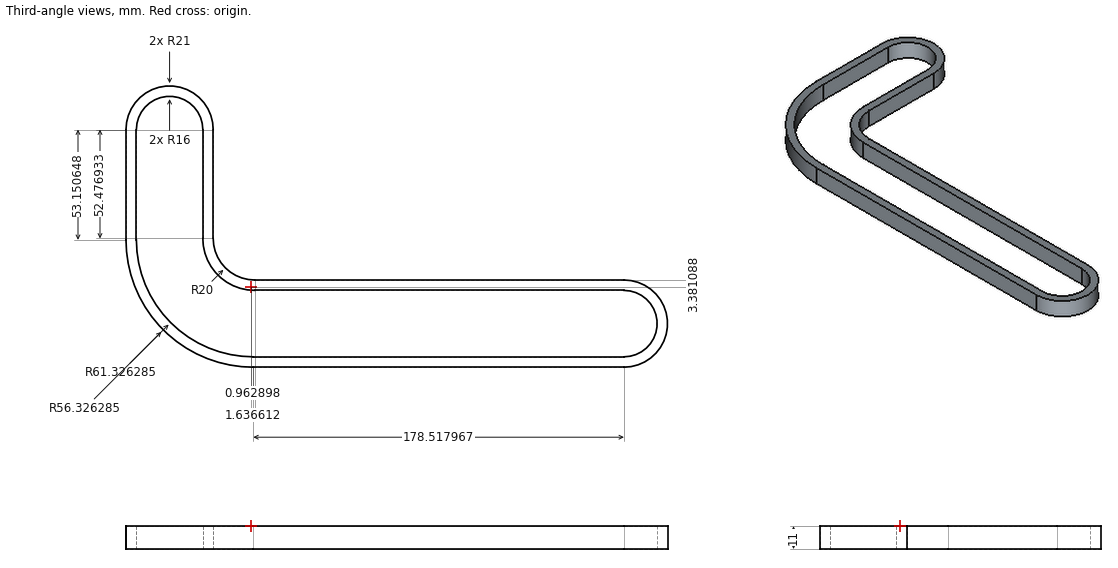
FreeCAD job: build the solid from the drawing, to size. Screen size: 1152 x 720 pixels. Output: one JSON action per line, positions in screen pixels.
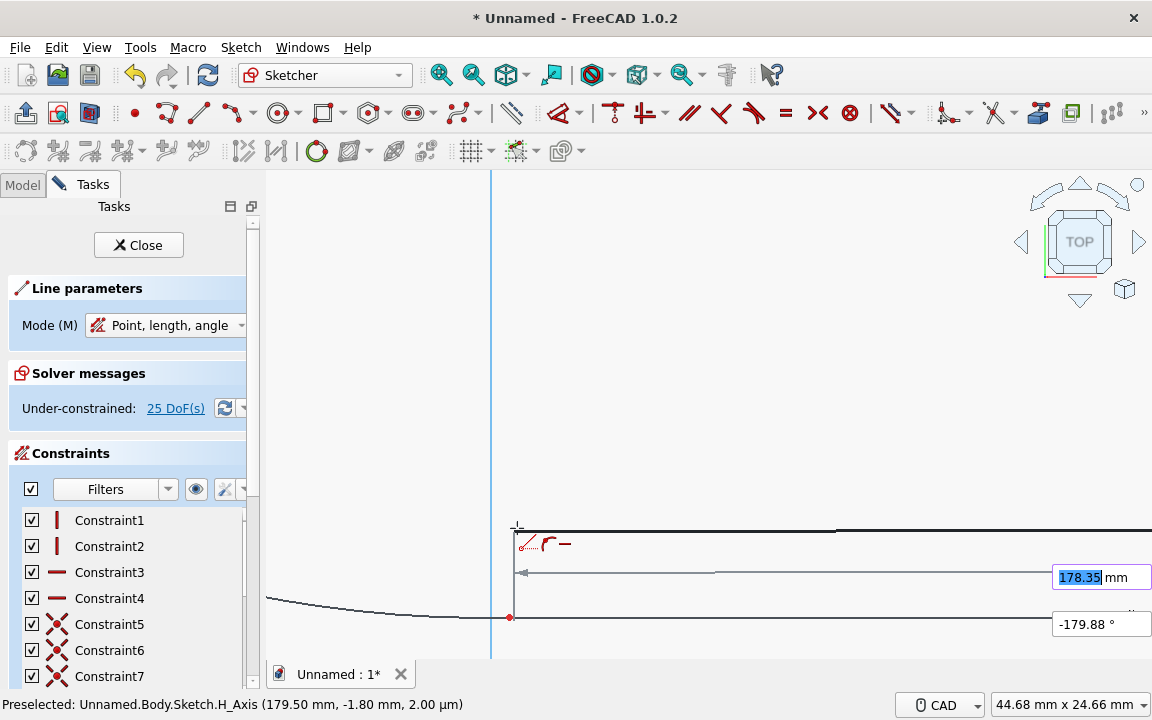
{"action": "left_click", "coordinate": [510, 518]}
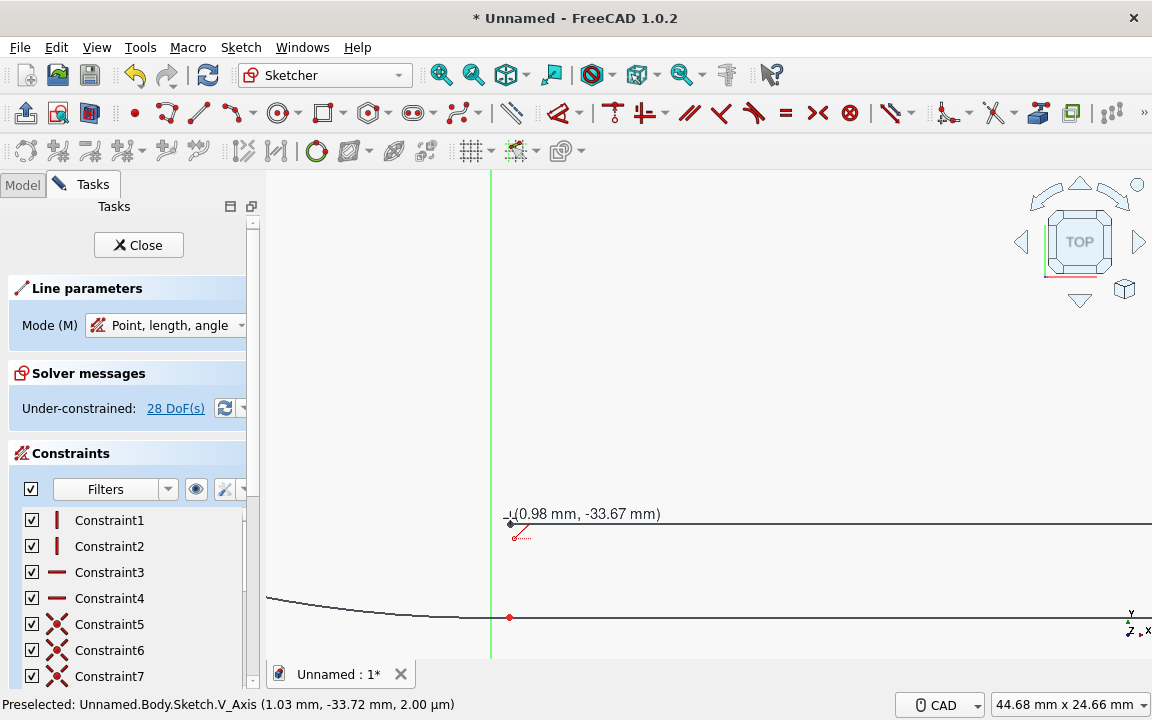
{"action": "left_click", "coordinate": [232, 114]}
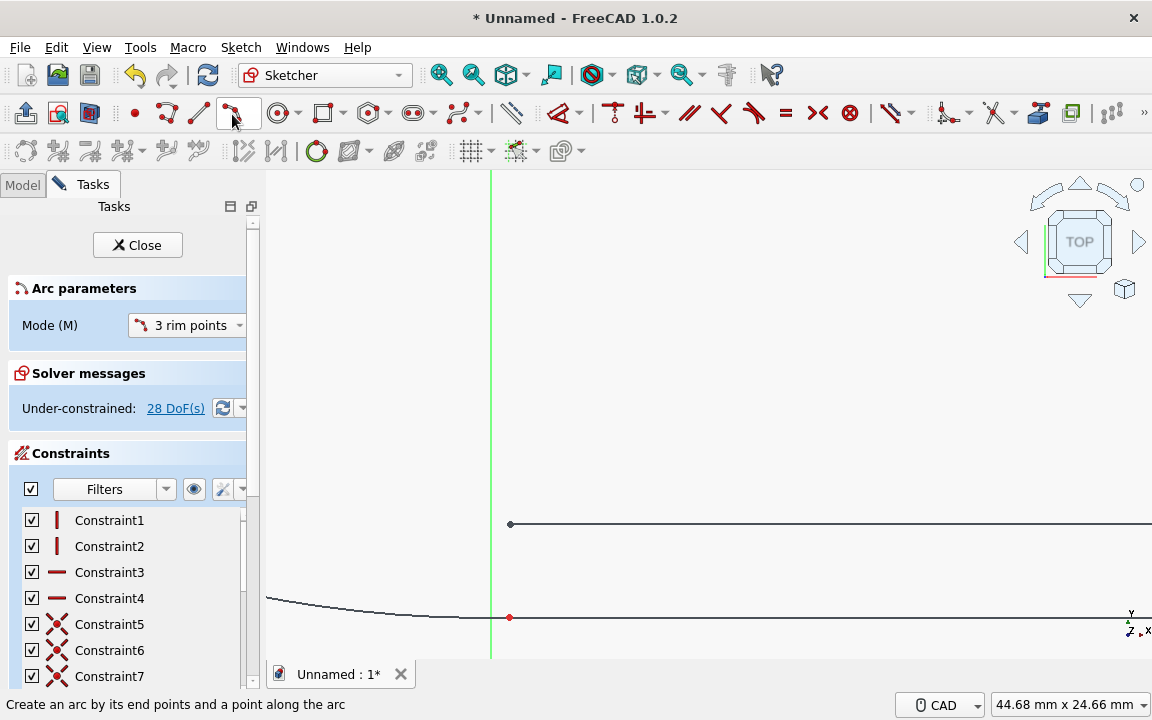
{"action": "scroll", "coordinate": [517, 528], "scroll_direction": "down", "scroll_amount": 12}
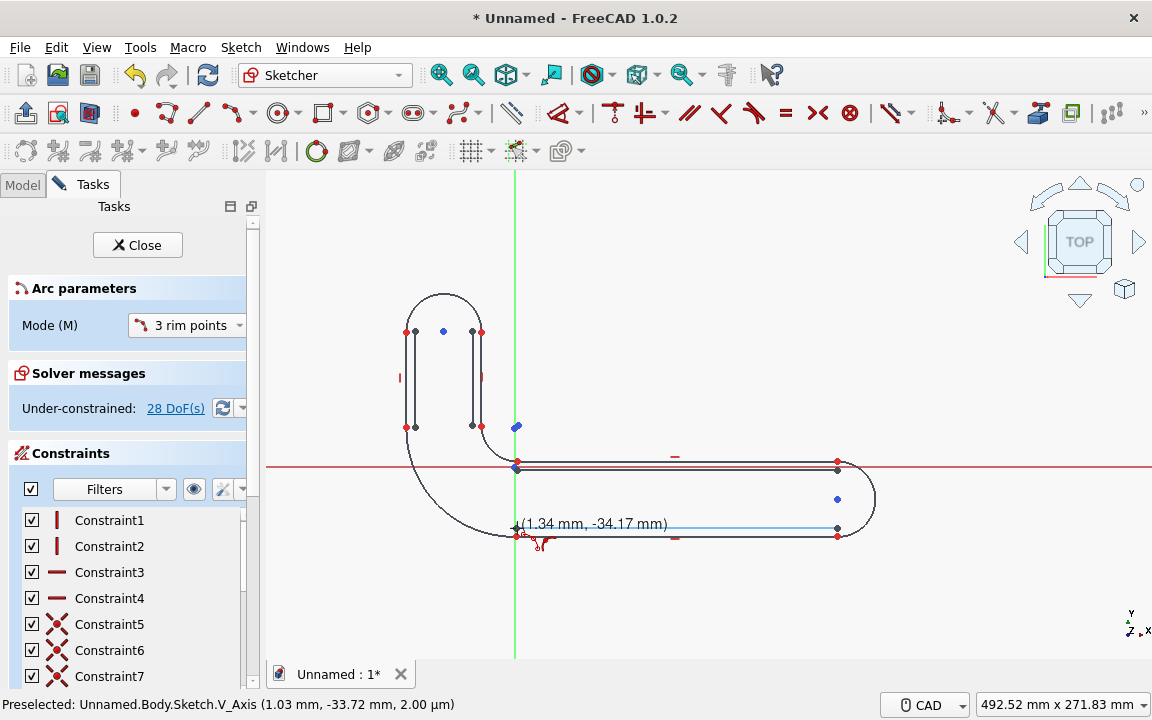
{"action": "scroll", "coordinate": [415, 331], "scroll_direction": "up", "scroll_amount": 3}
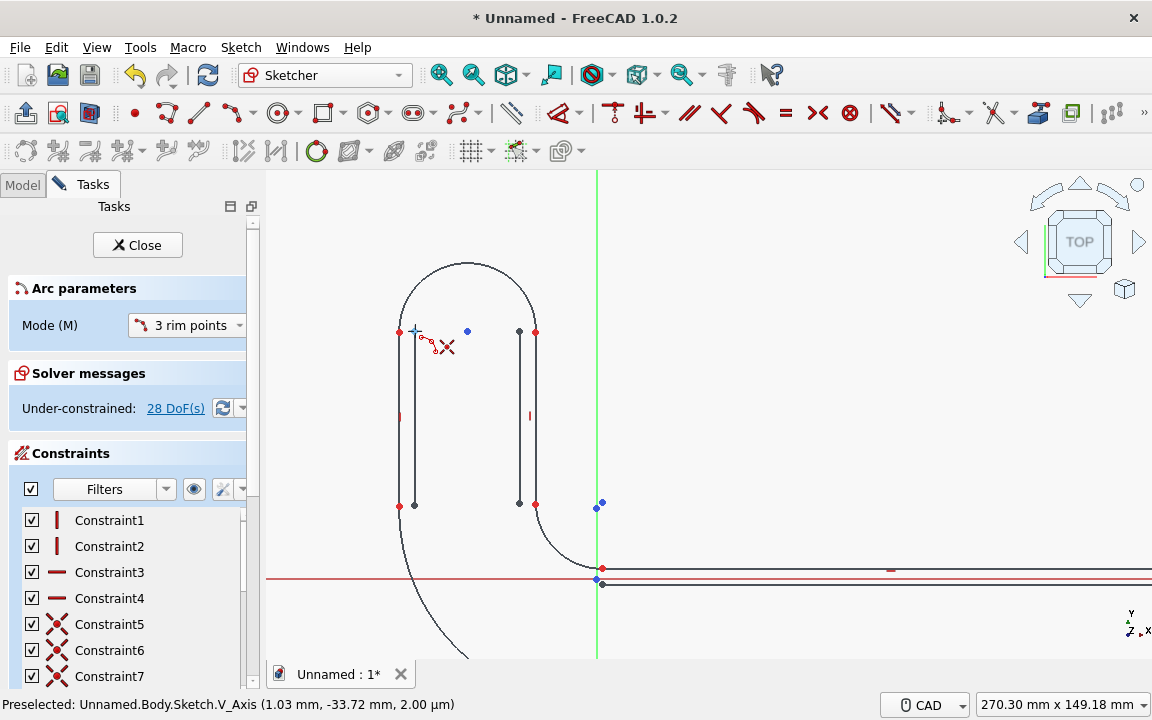
{"action": "left_click", "coordinate": [415, 332]}
{"action": "left_click", "coordinate": [520, 332]}
{"action": "left_click", "coordinate": [437, 288]}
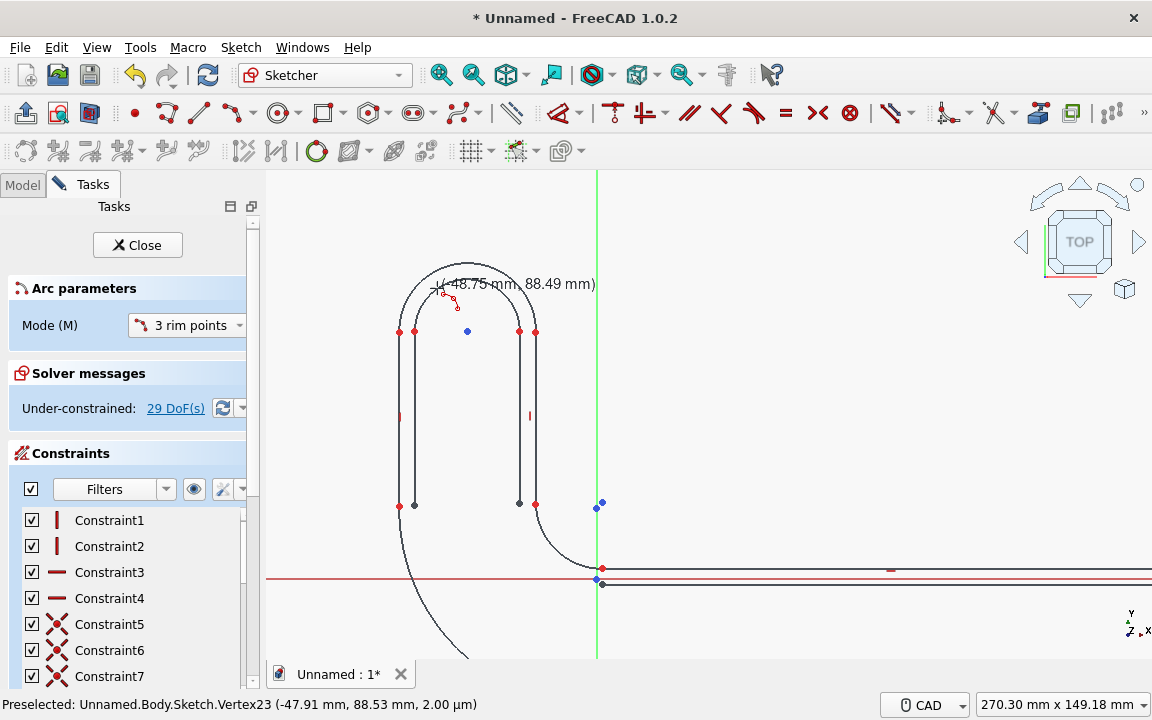
{"action": "left_click", "coordinate": [520, 504]}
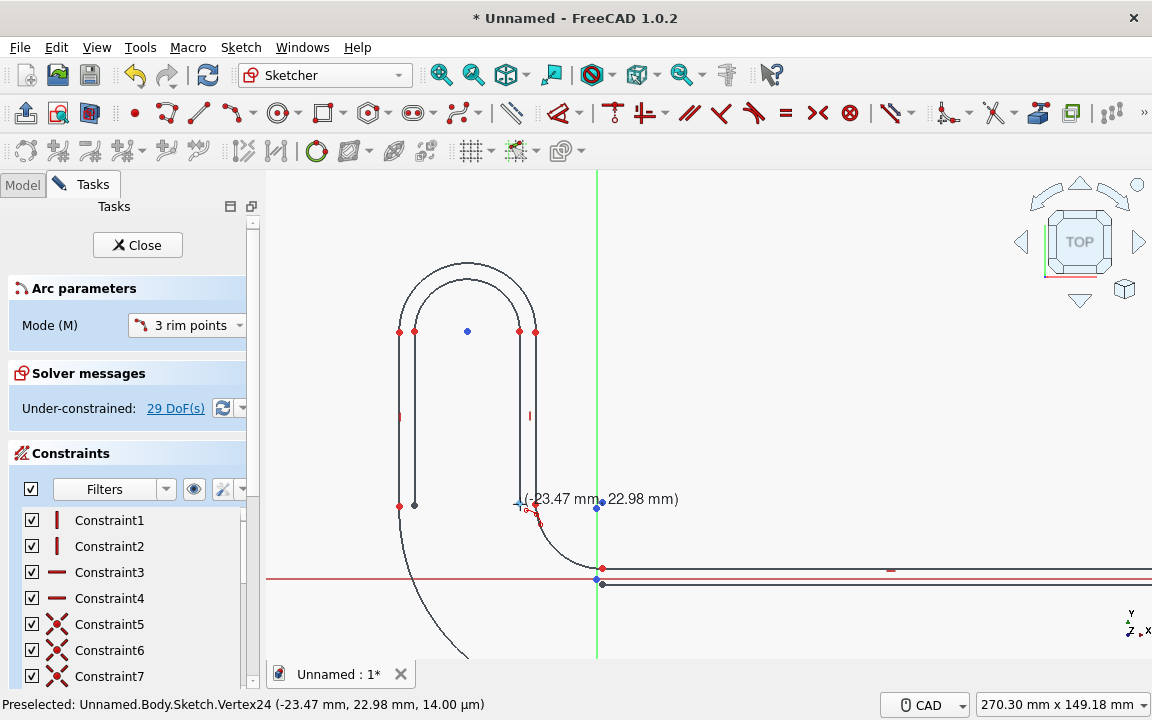
{"action": "scroll", "coordinate": [602, 584], "scroll_direction": "up", "scroll_amount": 6}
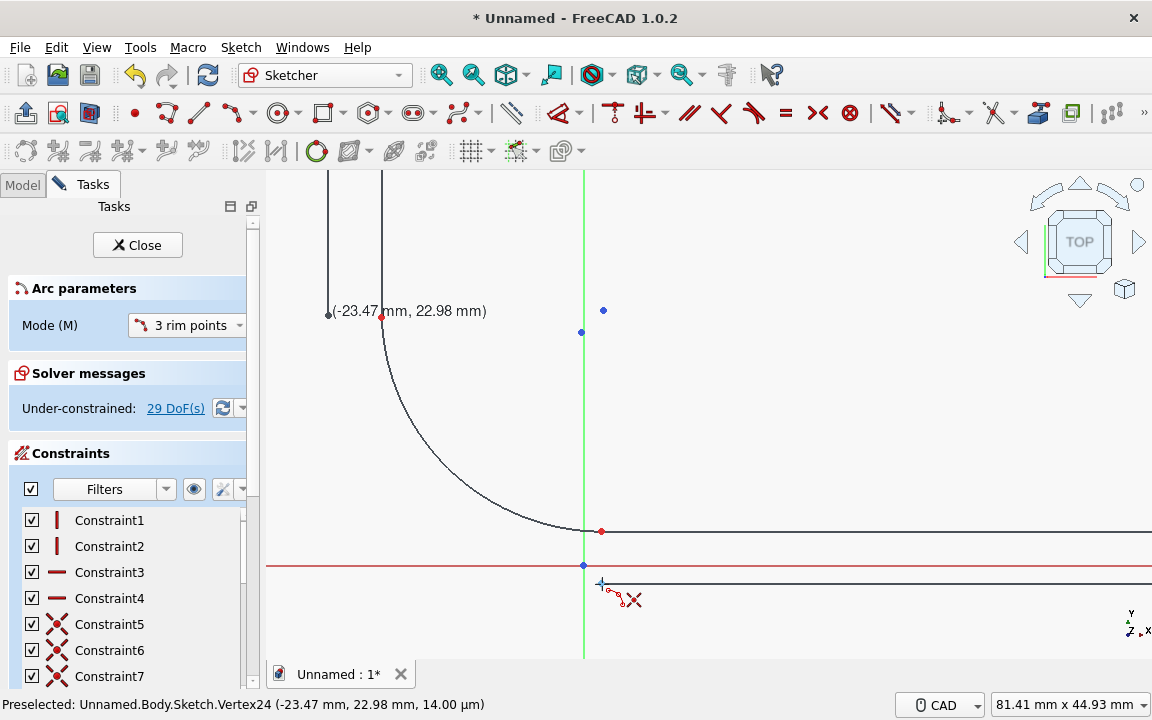
{"action": "left_click", "coordinate": [601, 584]}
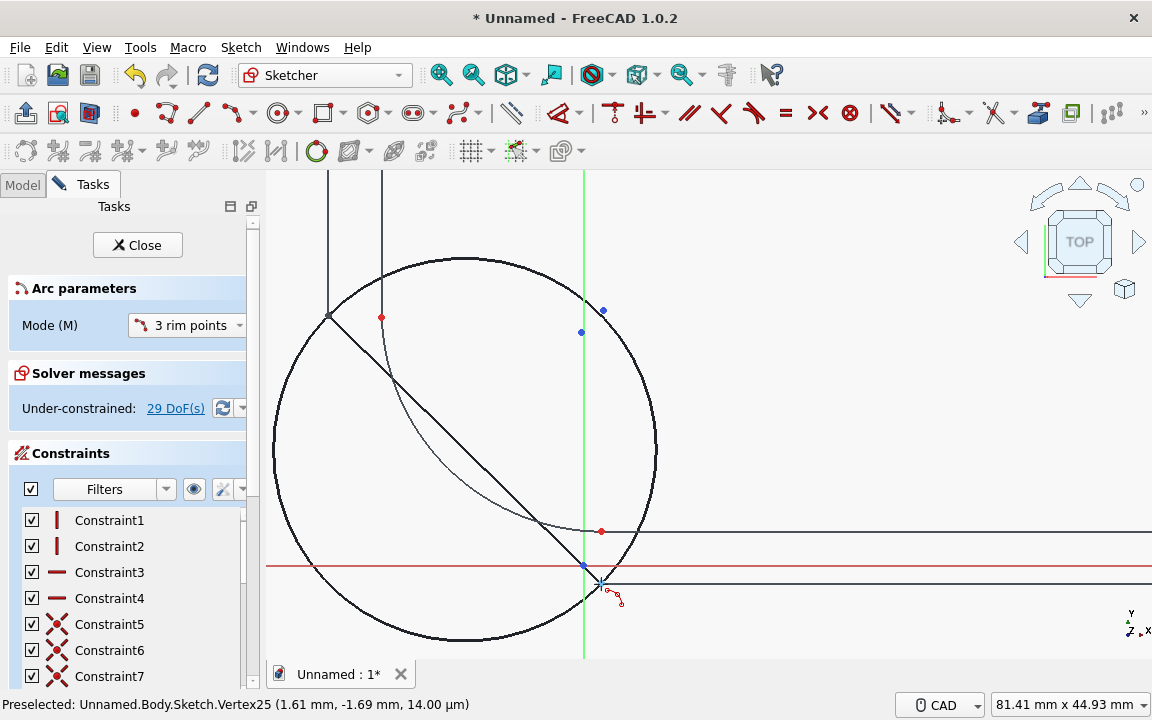
{"action": "scroll", "coordinate": [501, 447], "scroll_direction": "down", "scroll_amount": 9}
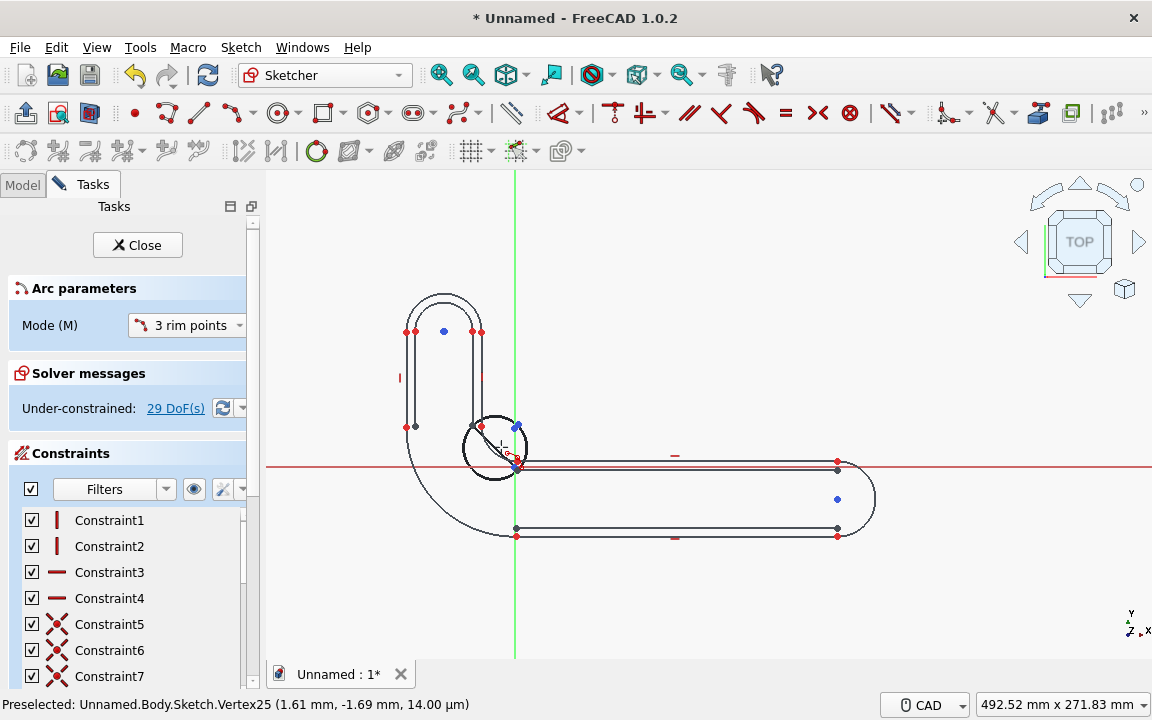
{"action": "scroll", "coordinate": [478, 445], "scroll_direction": "up", "scroll_amount": 3}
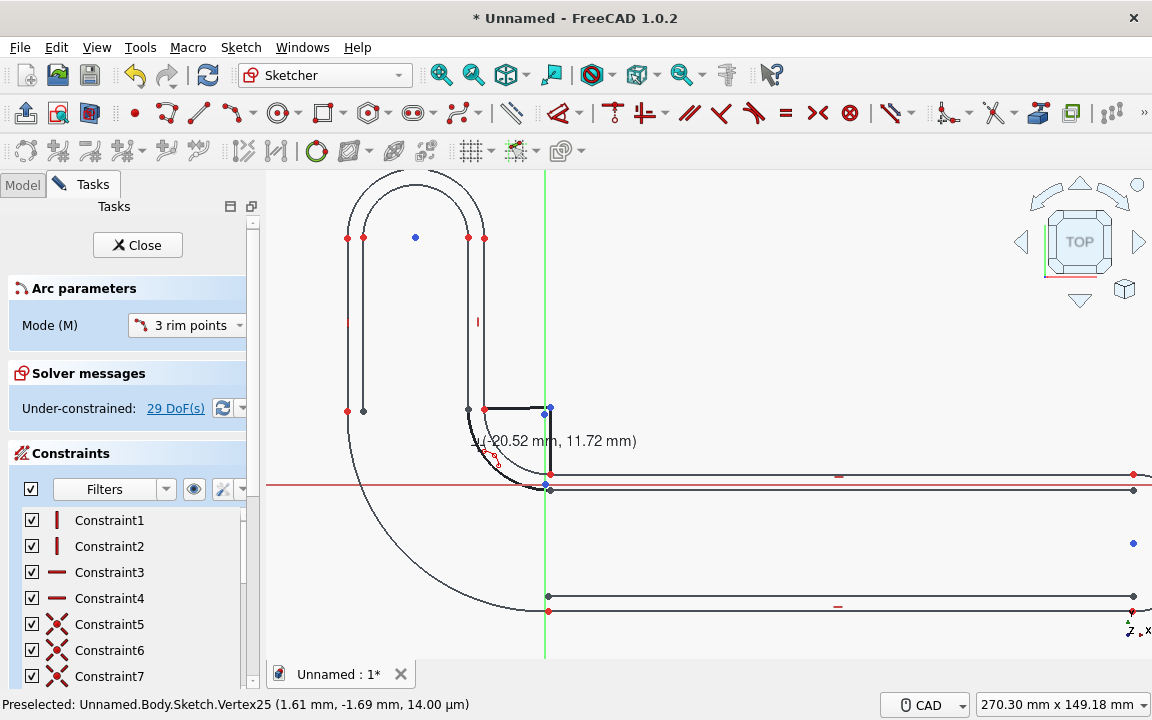
{"action": "left_click", "coordinate": [477, 445]}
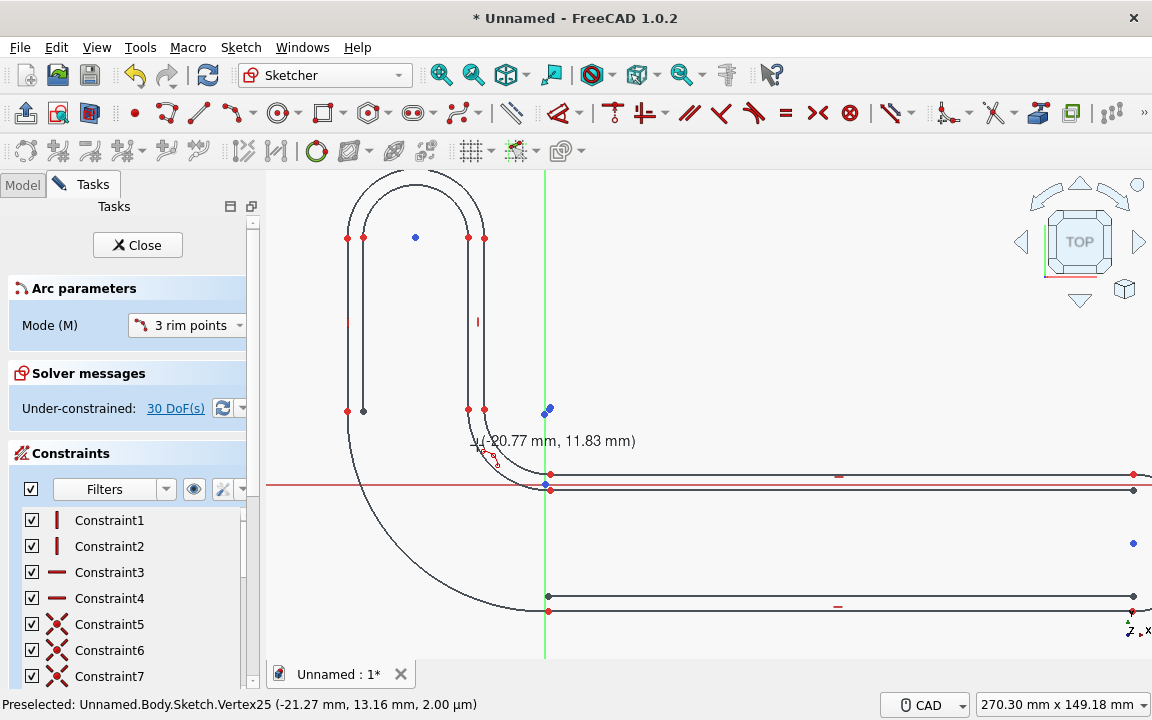
{"action": "scroll", "coordinate": [477, 445], "scroll_direction": "down", "scroll_amount": 3}